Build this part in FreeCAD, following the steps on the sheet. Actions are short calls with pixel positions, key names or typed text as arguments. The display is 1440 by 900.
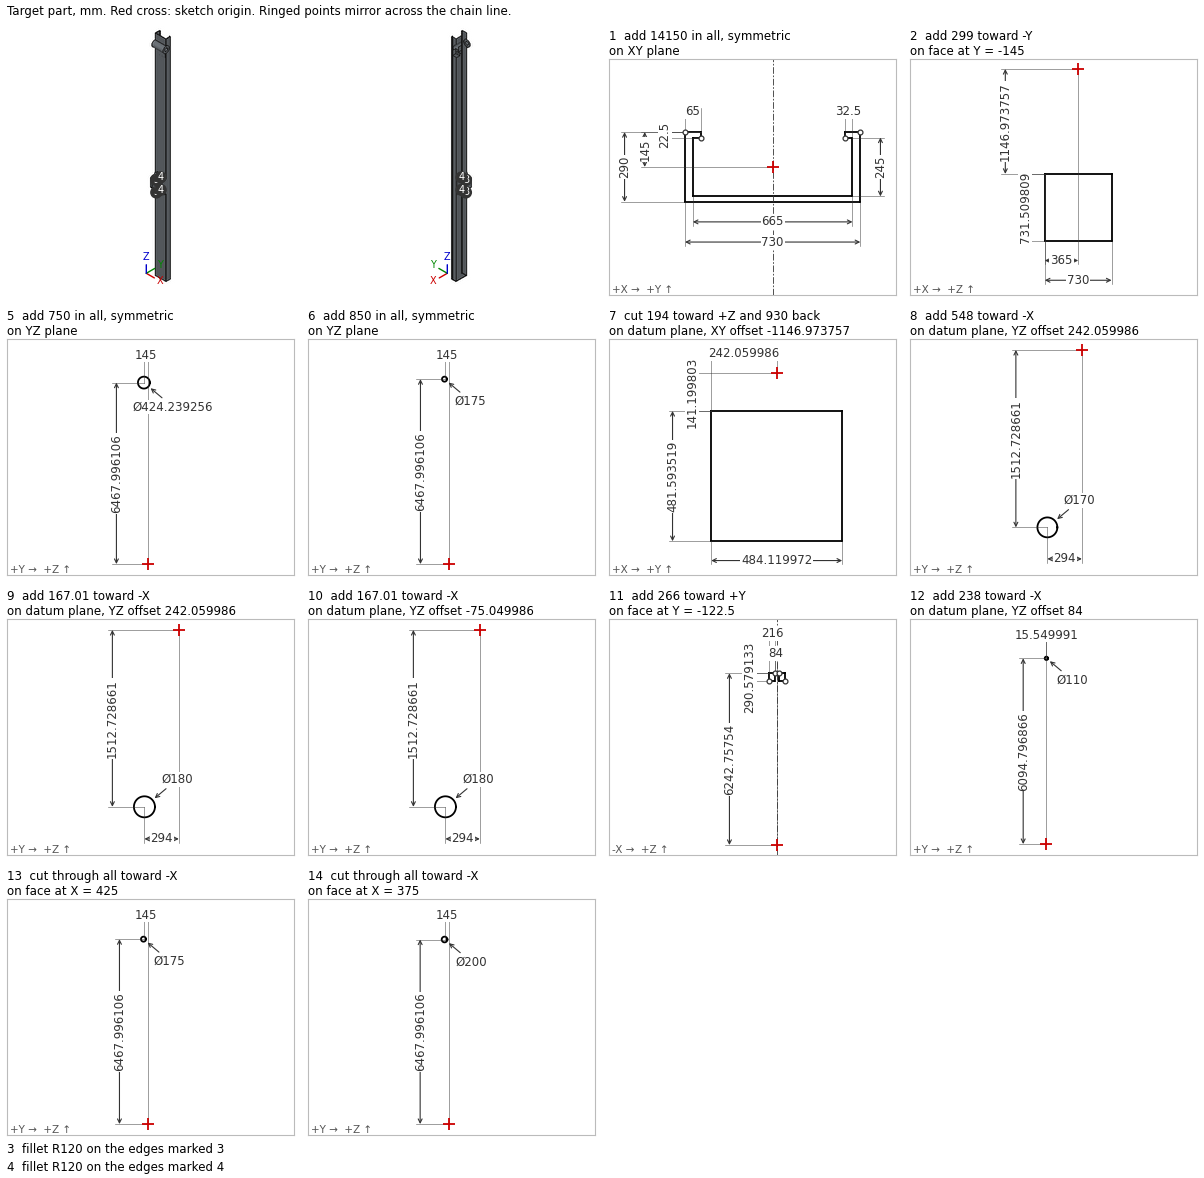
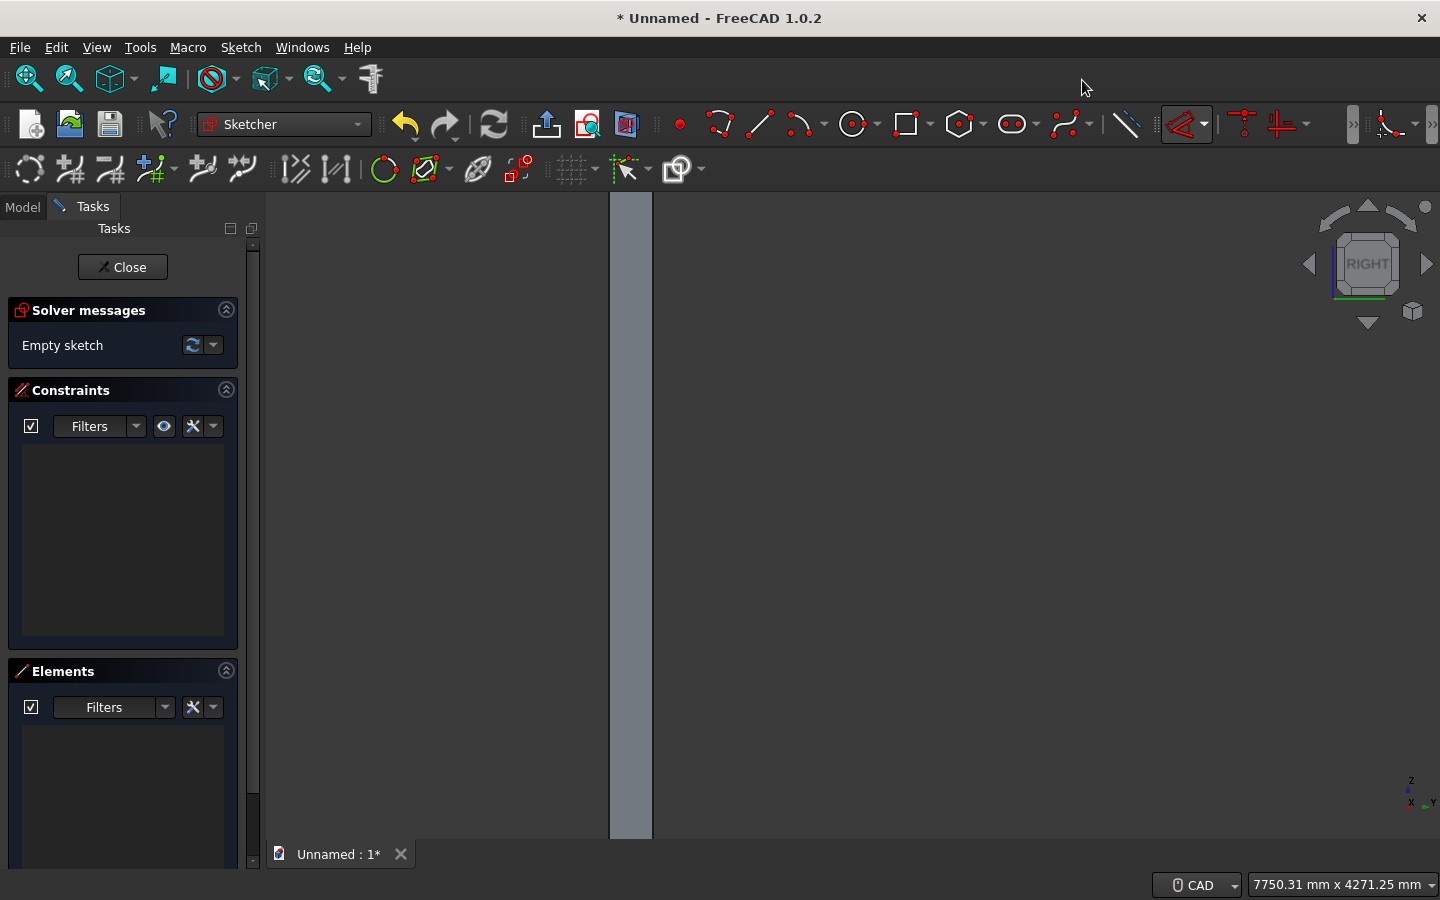
scroll(784, 516, down, 5)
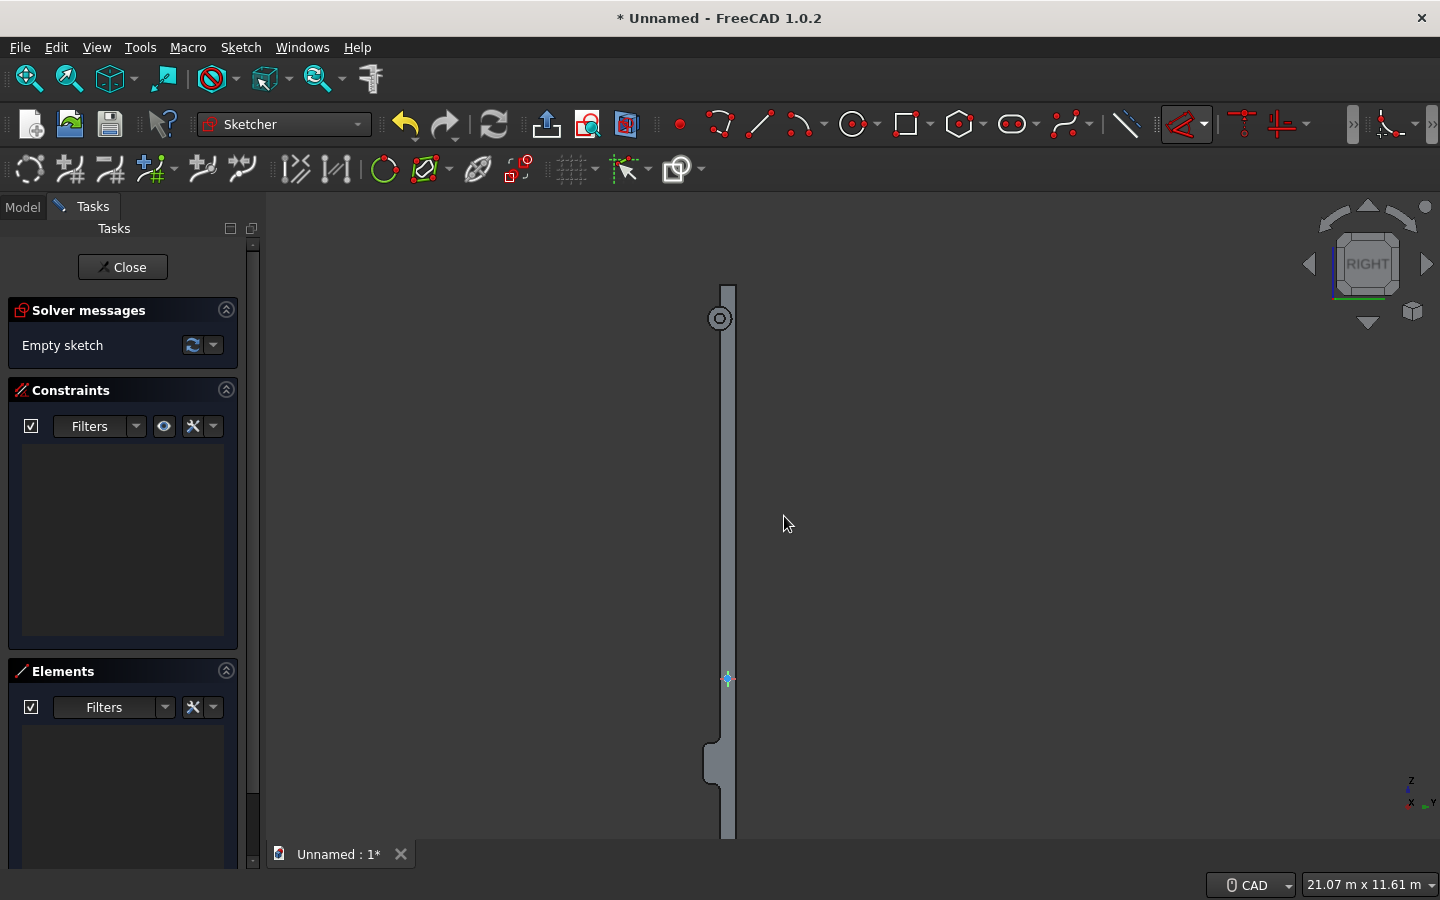
scroll(716, 308, up, 15)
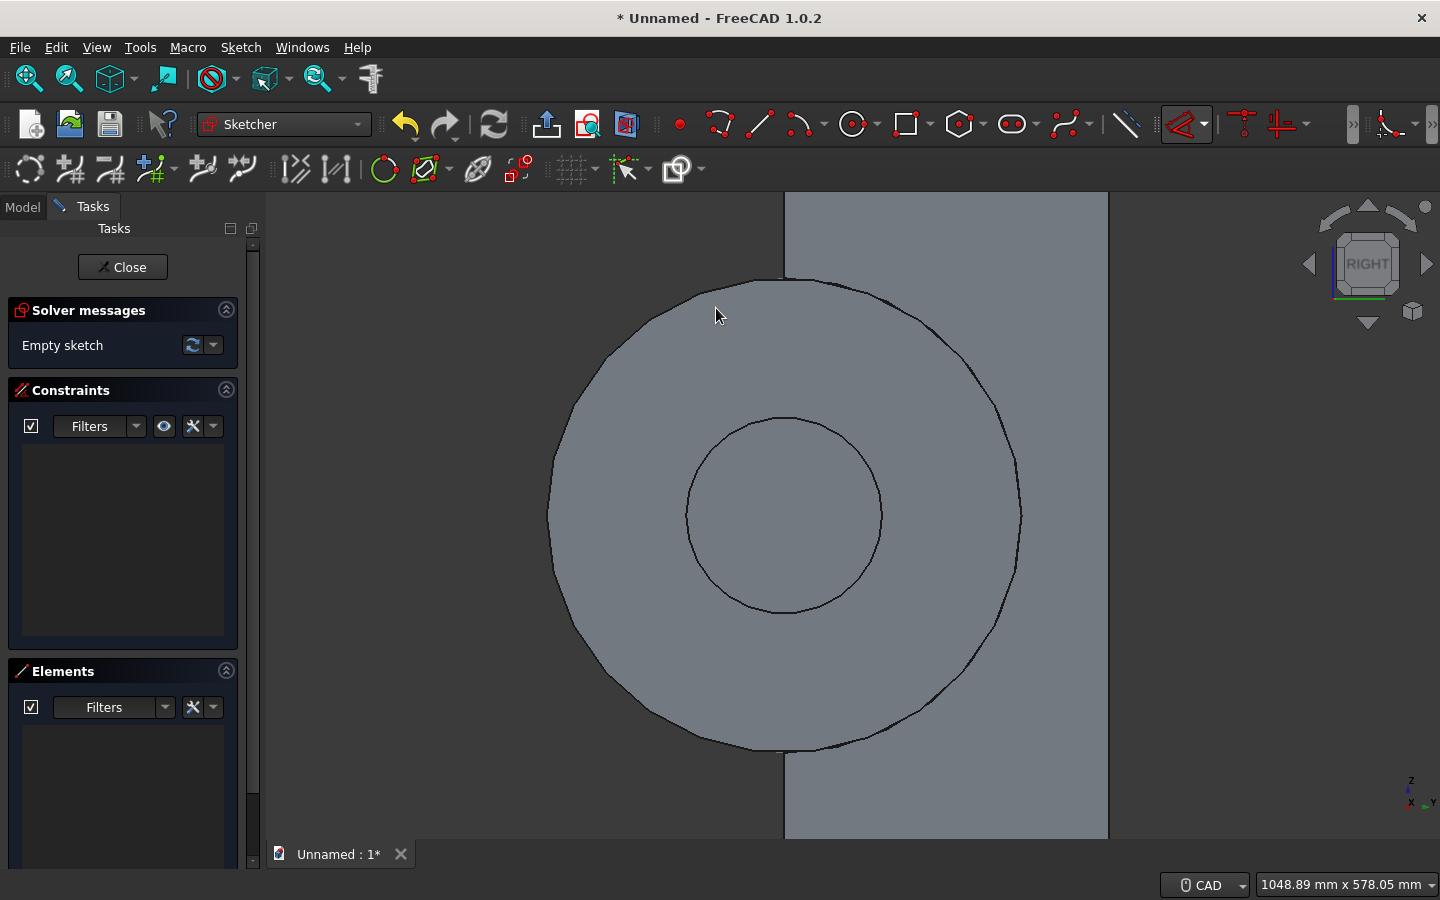
scroll(784, 516, up, 4)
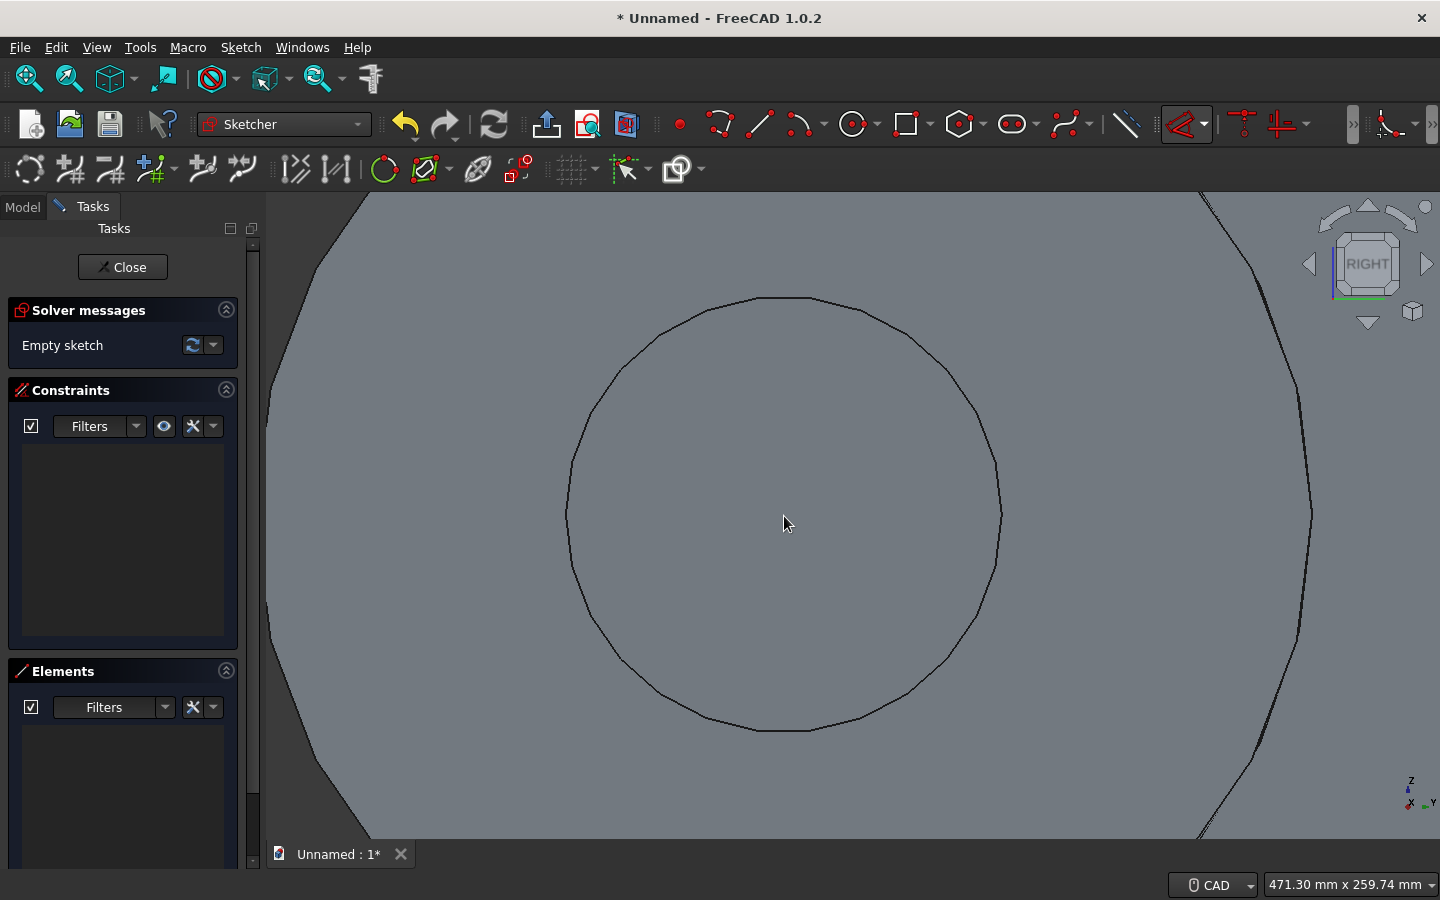
key(g)
key(c)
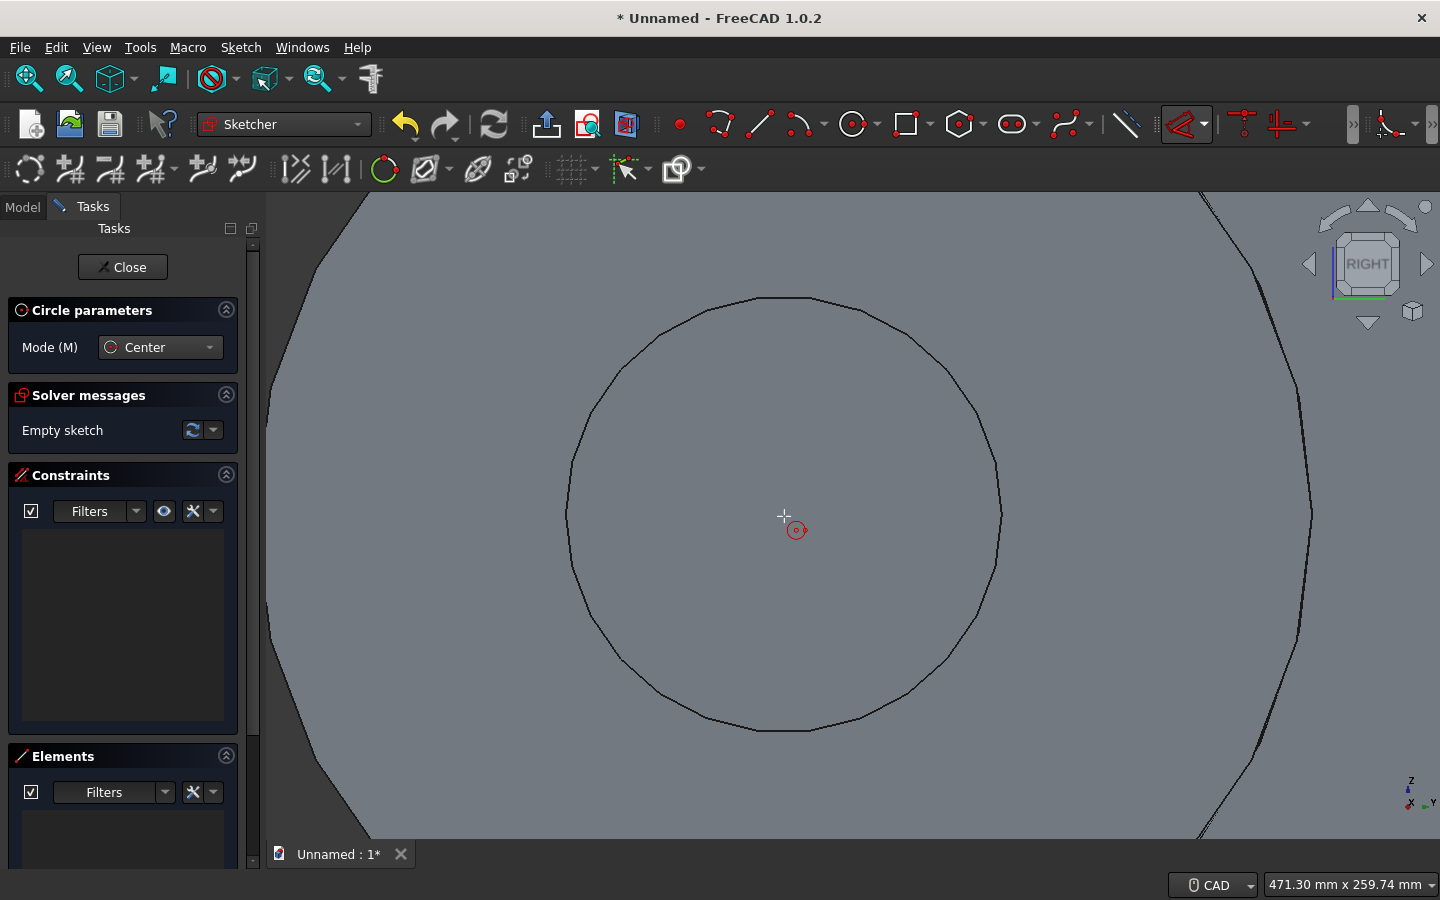
click(784, 514)
click(938, 360)
key(Escape)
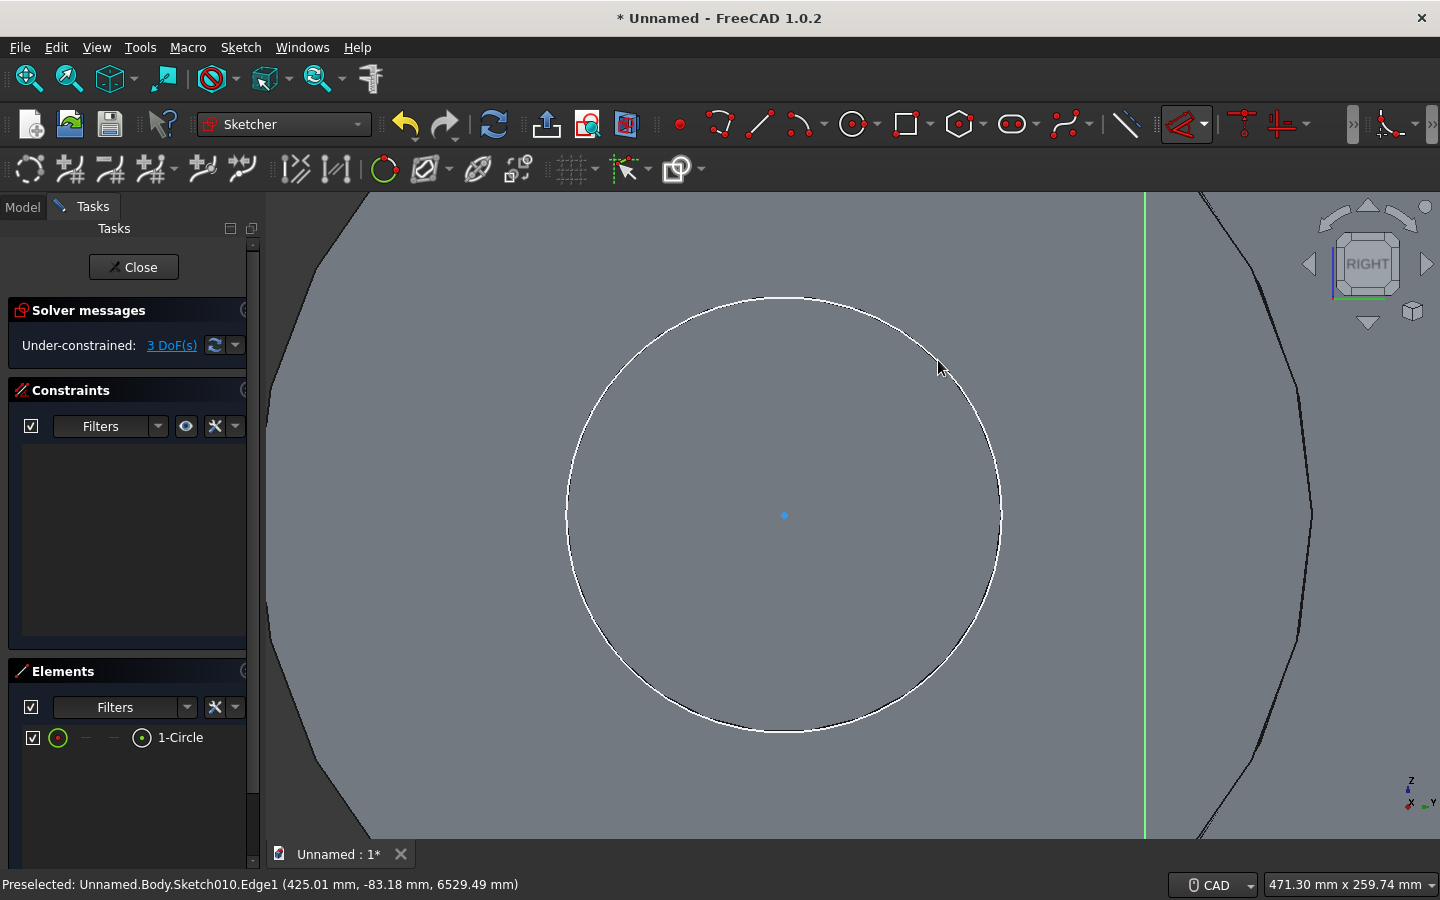
click(938, 361)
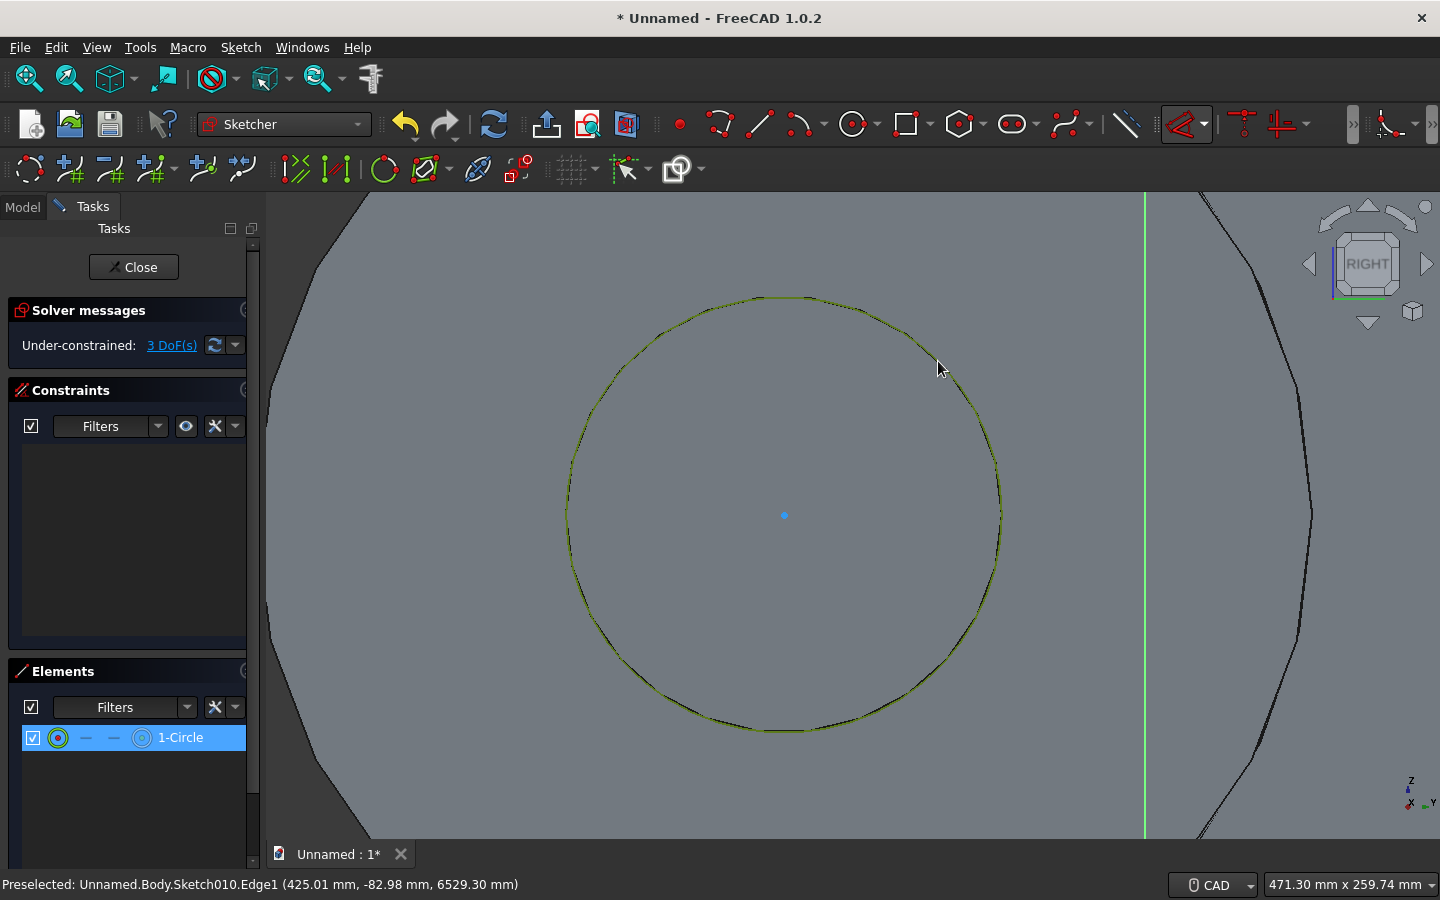
key(k)
key(o)